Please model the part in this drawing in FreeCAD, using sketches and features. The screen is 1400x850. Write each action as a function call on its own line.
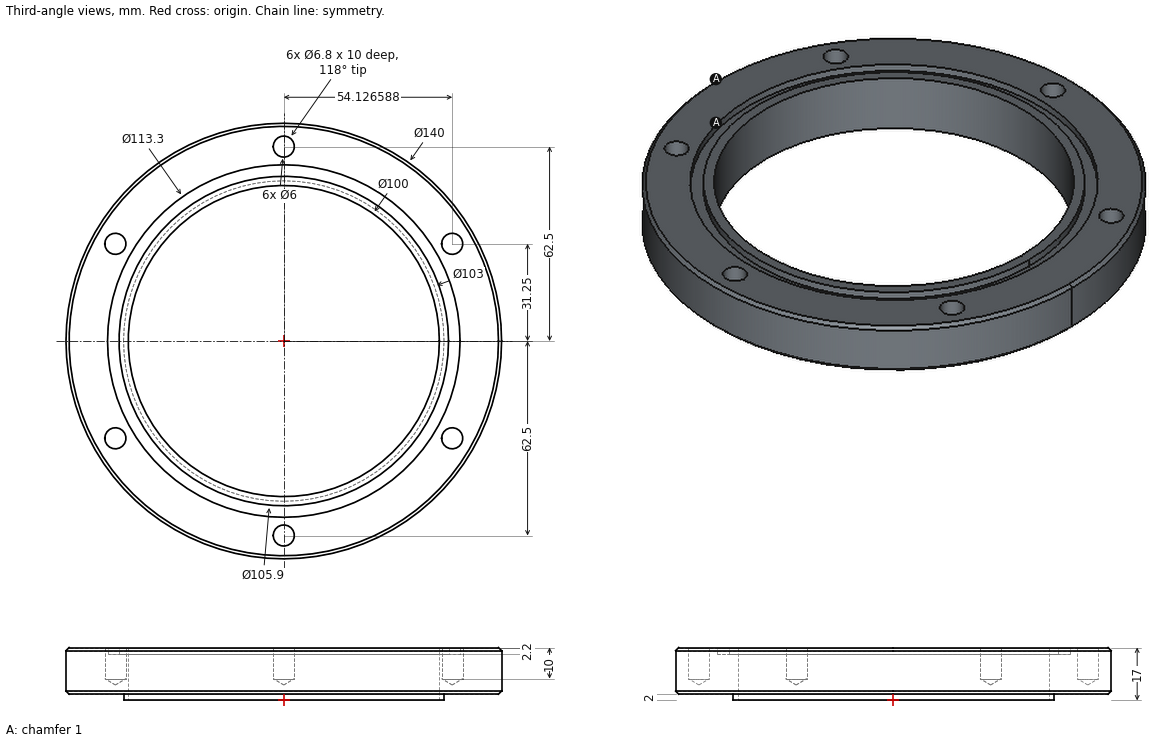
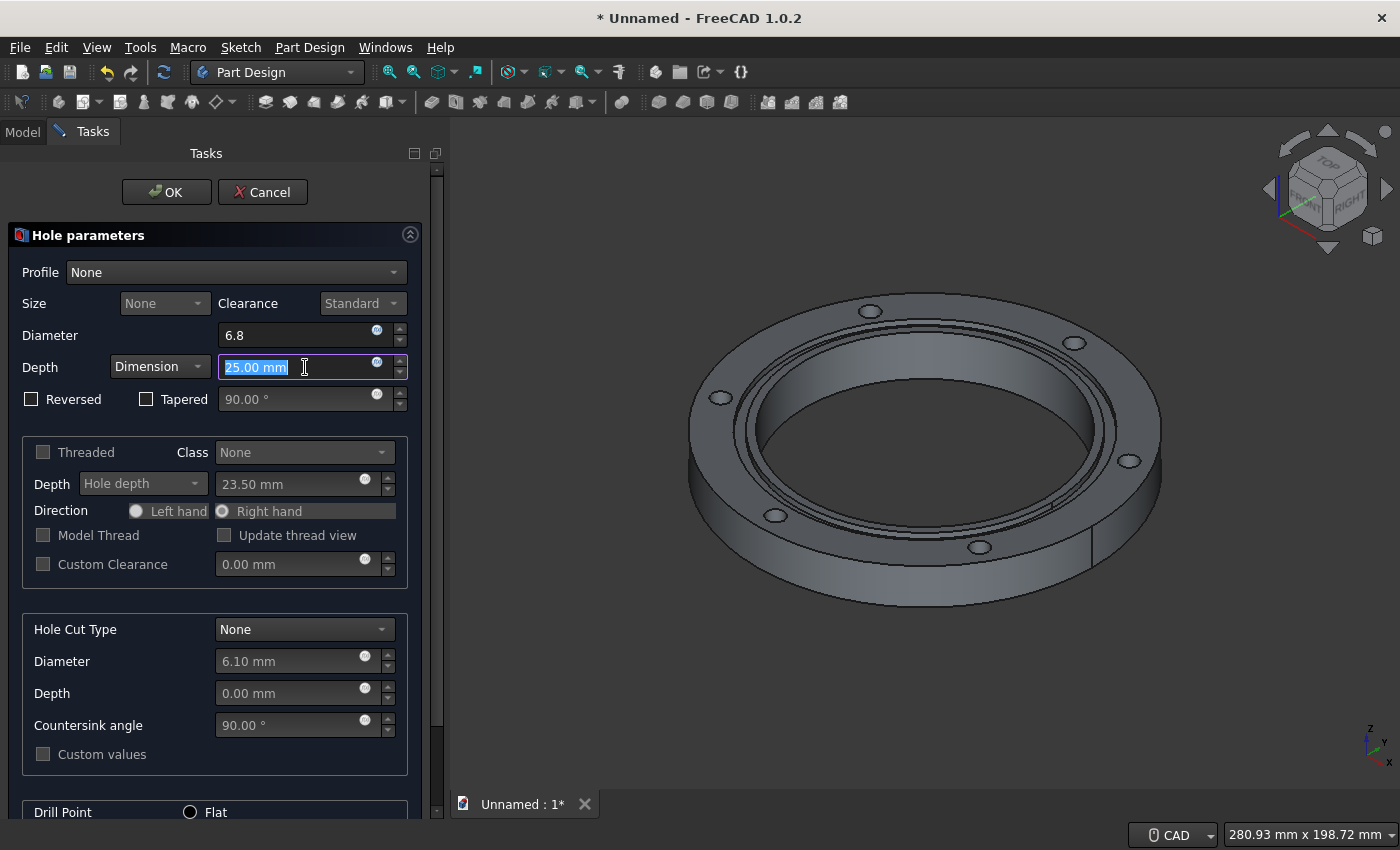
text(10)
key(Tab)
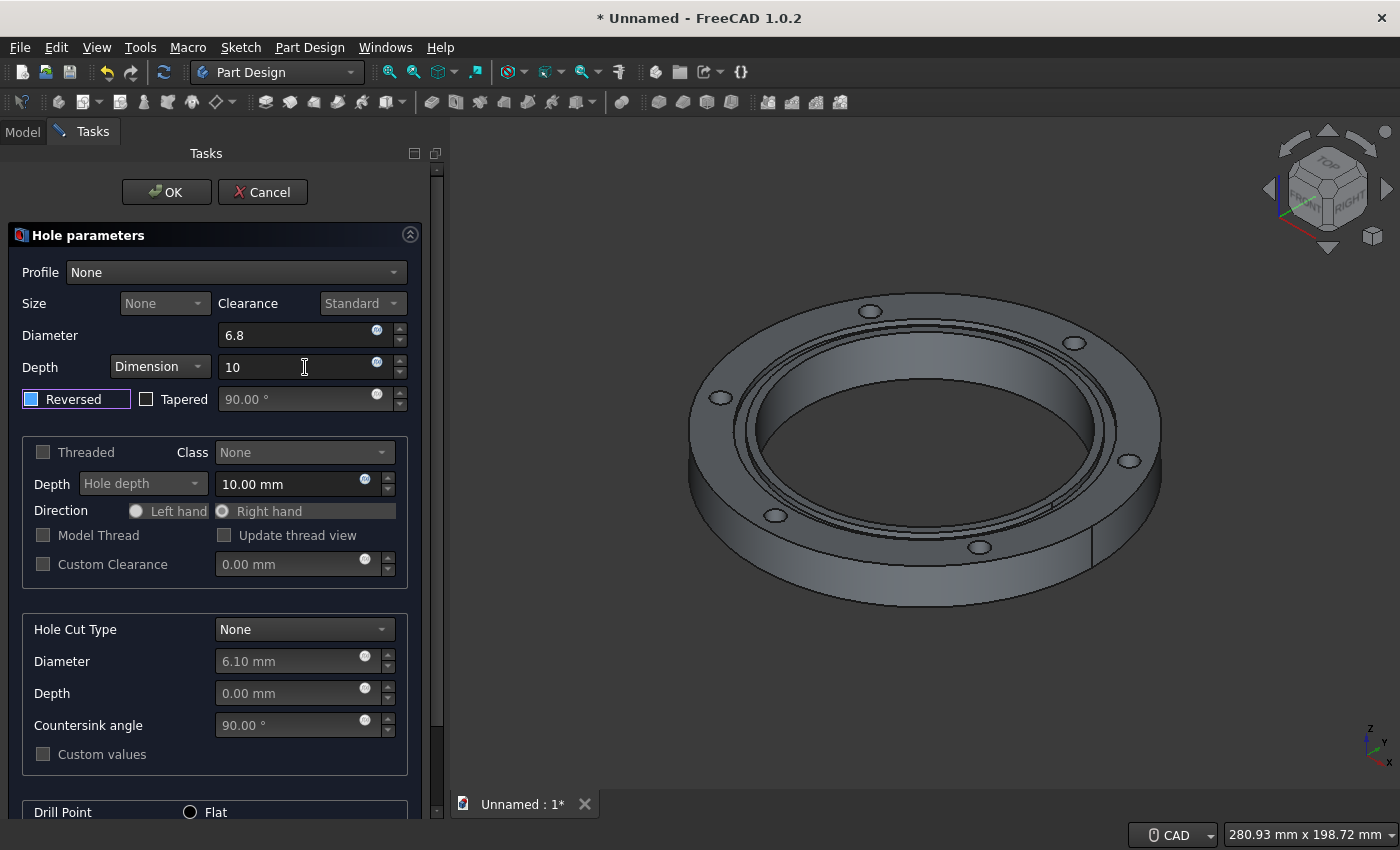
click(167, 192)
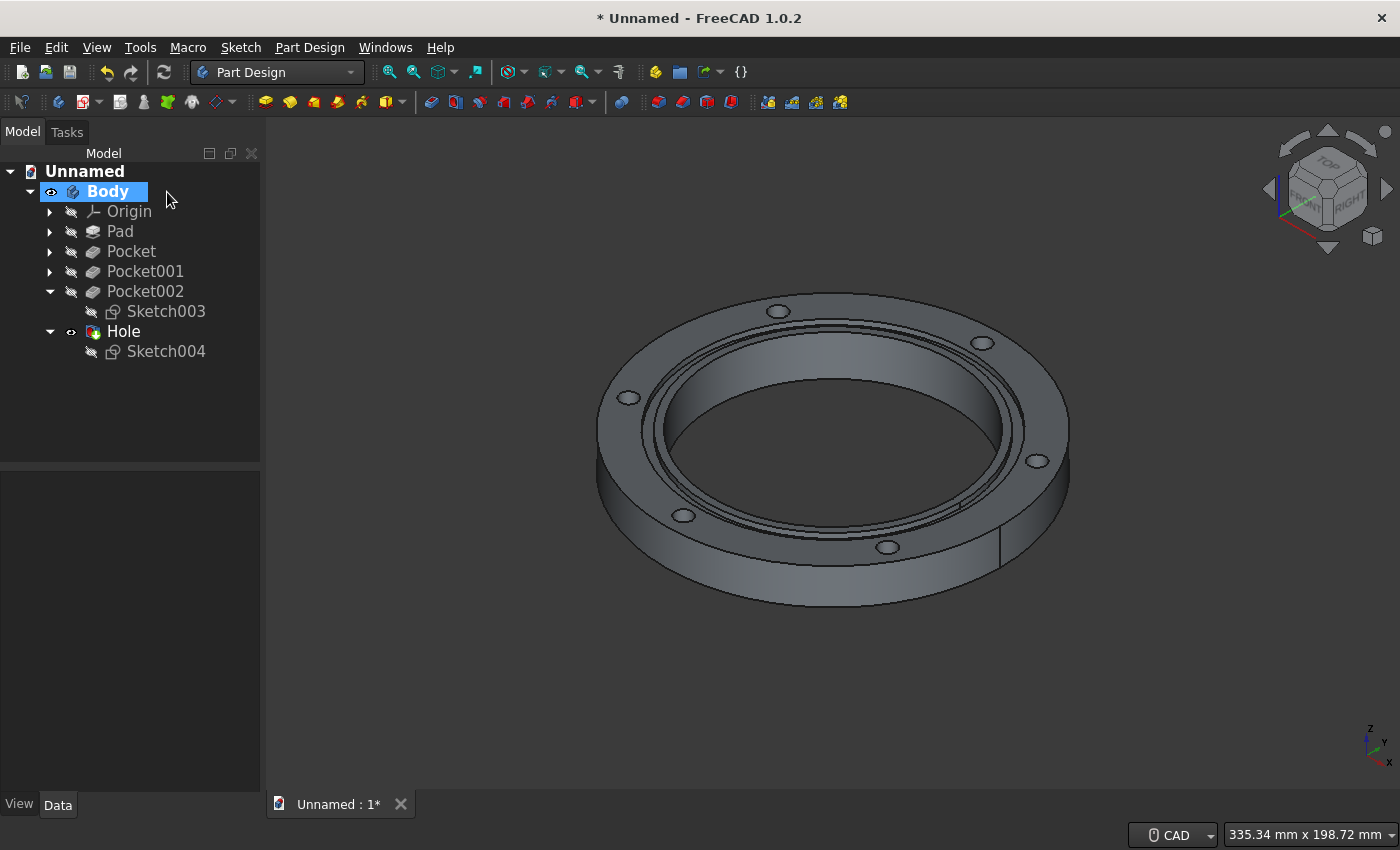
click(622, 491)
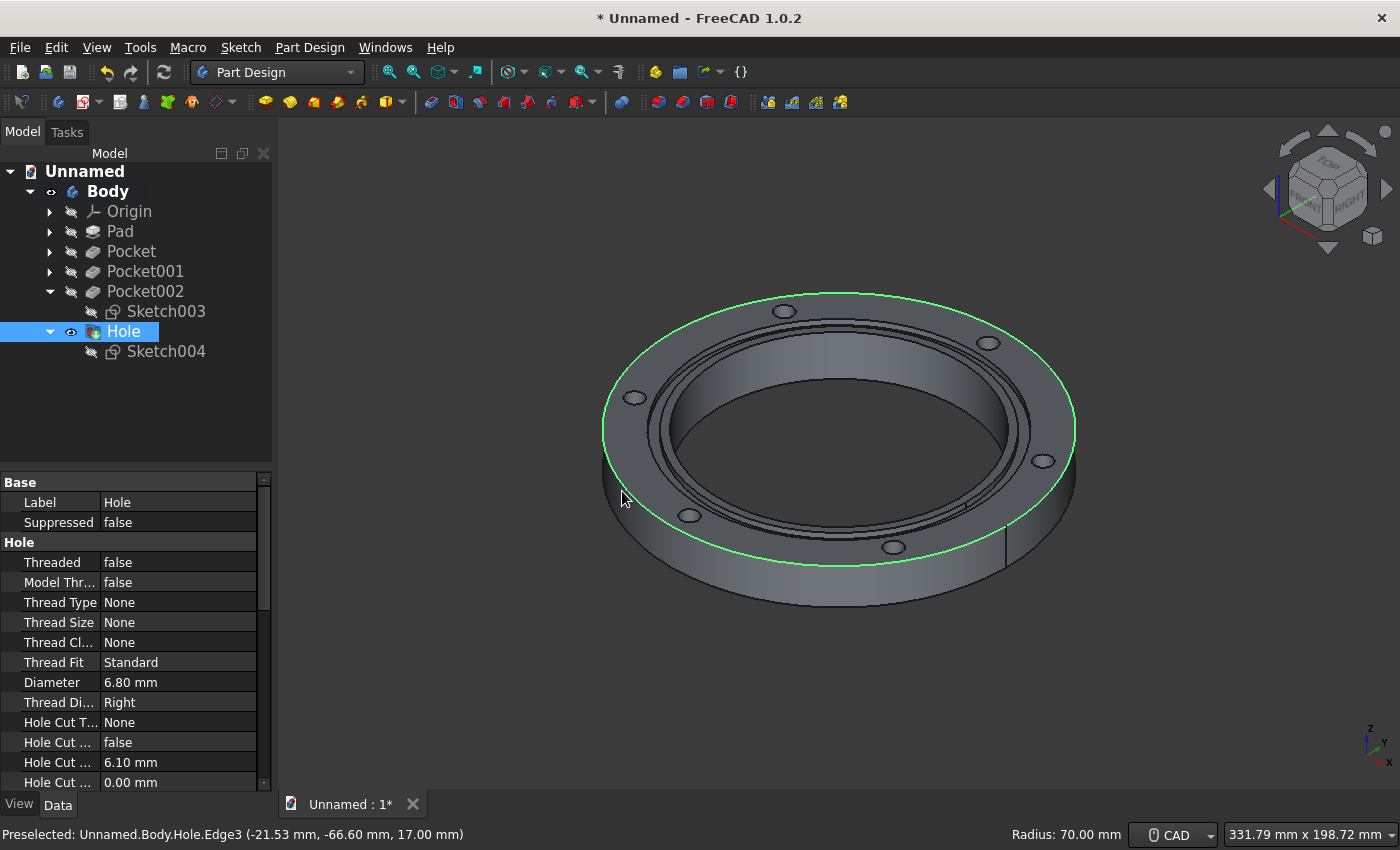
key(2)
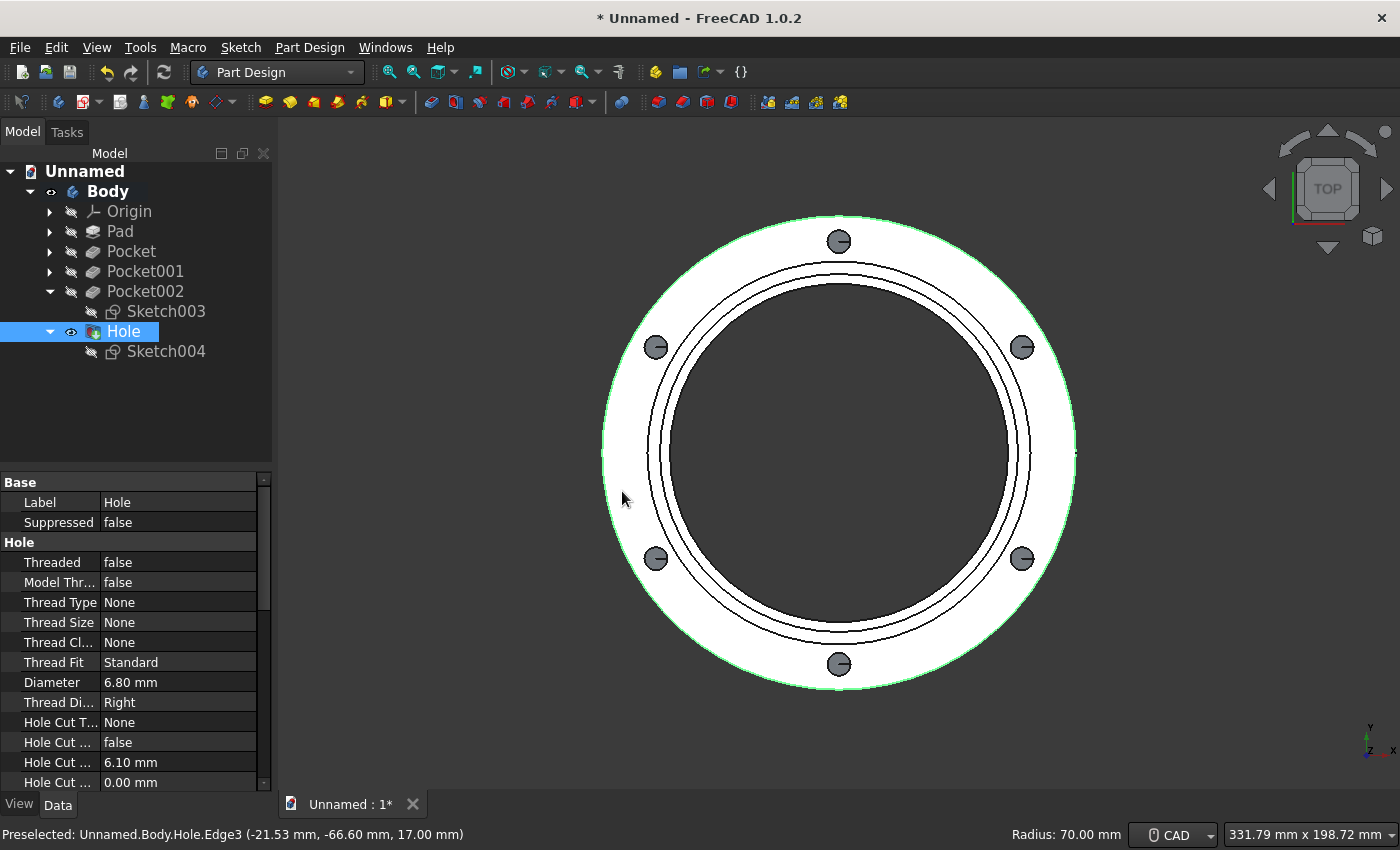
key(0)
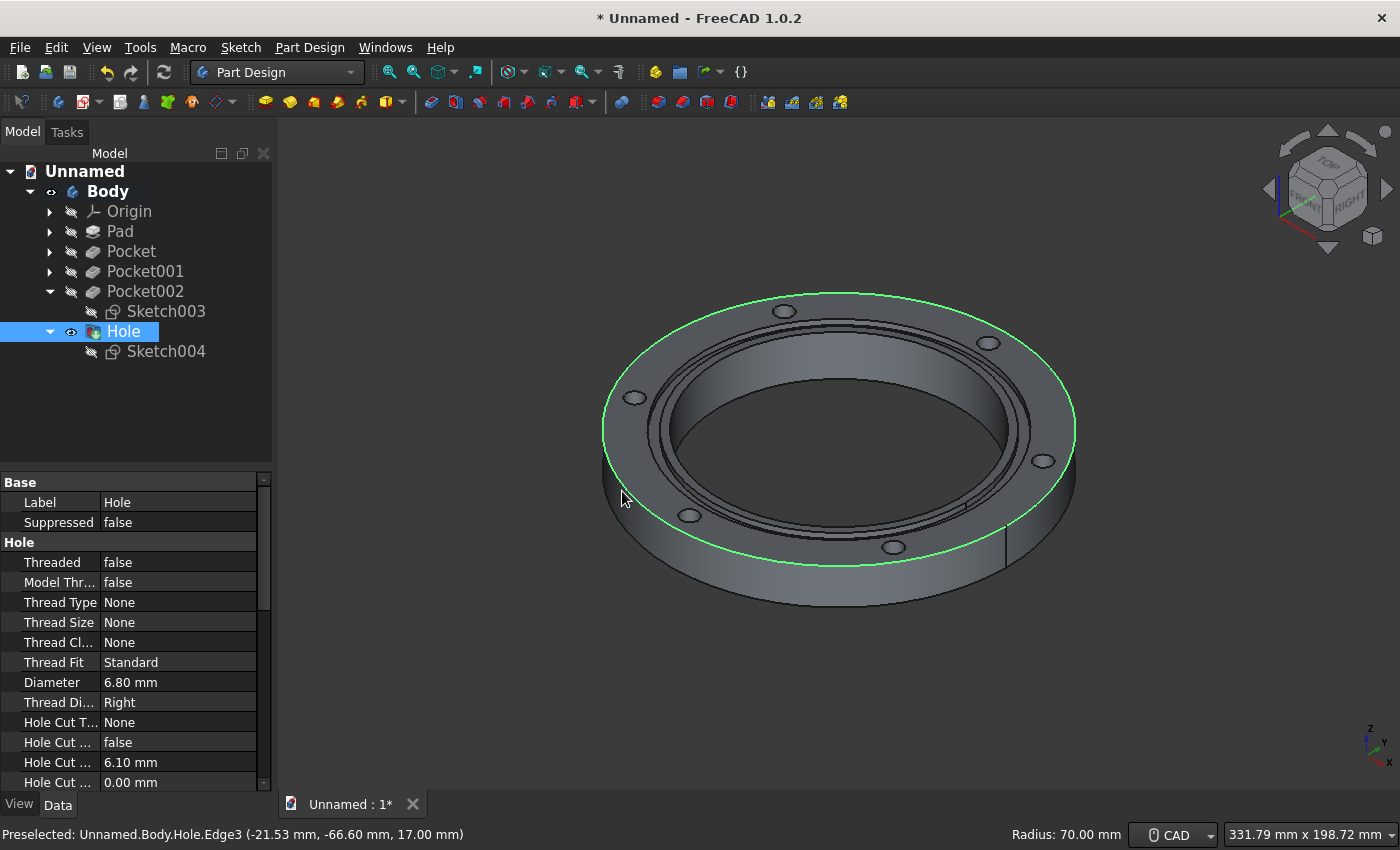
key(1)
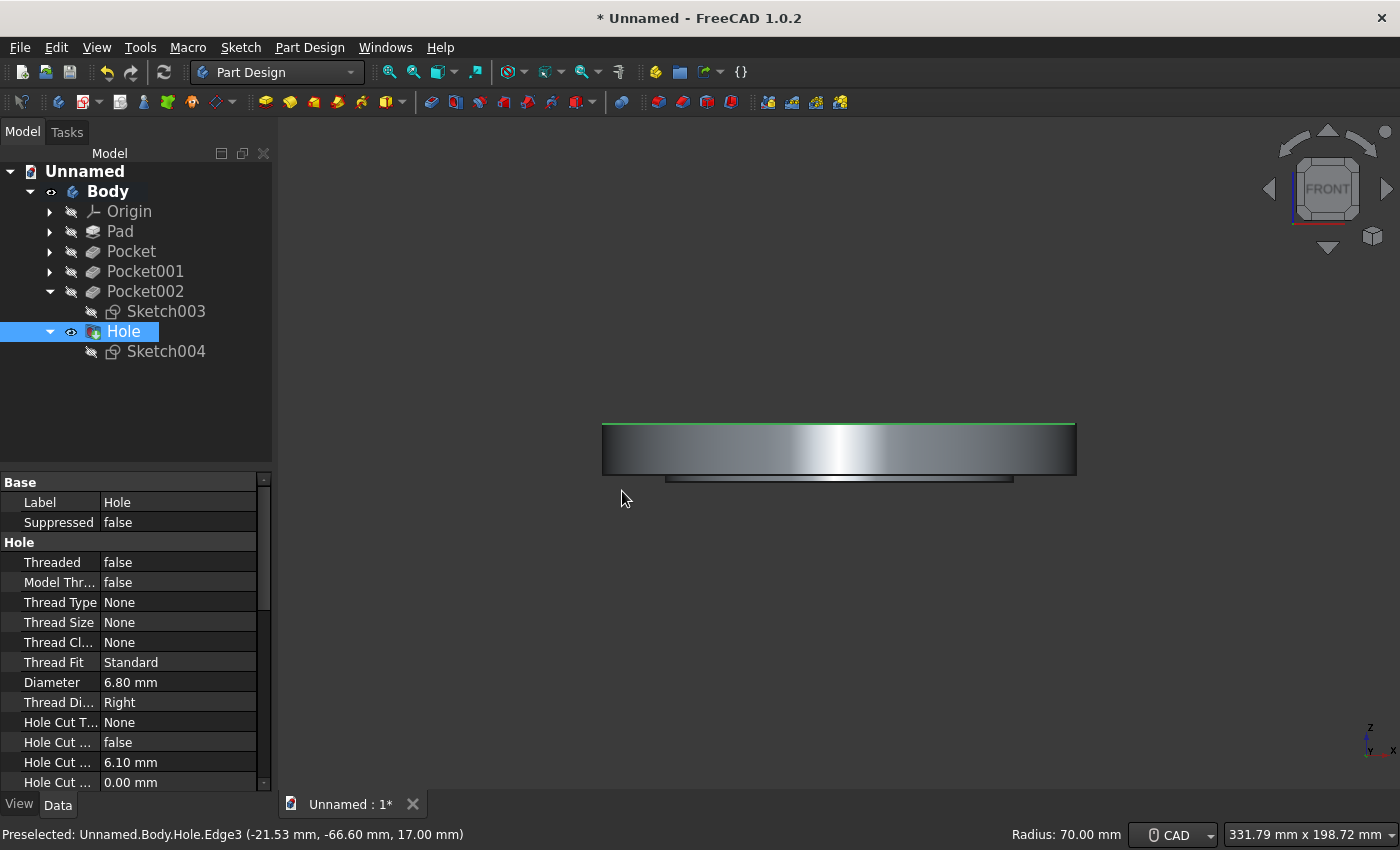
click(390, 72)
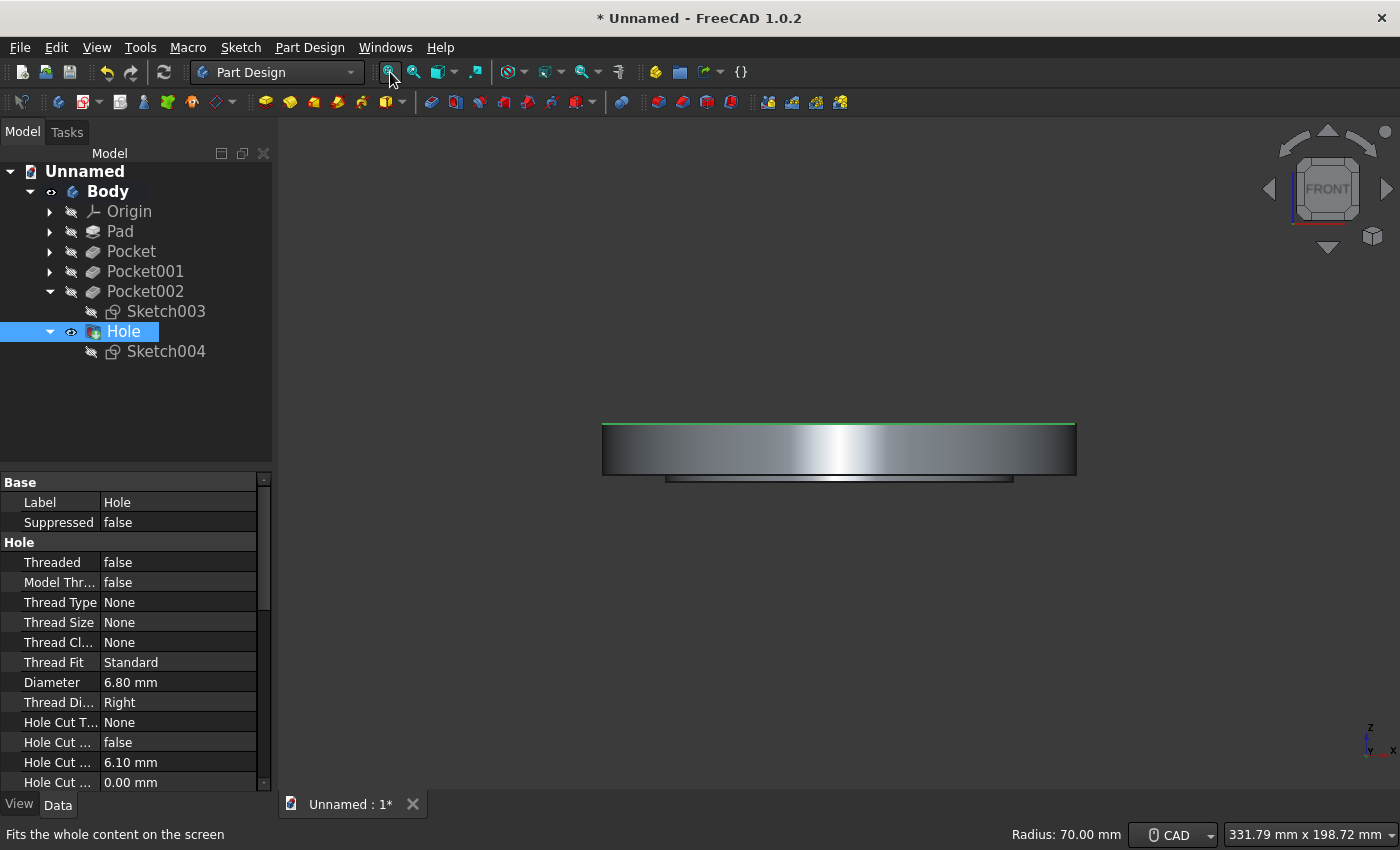
click(647, 474, ctrl)